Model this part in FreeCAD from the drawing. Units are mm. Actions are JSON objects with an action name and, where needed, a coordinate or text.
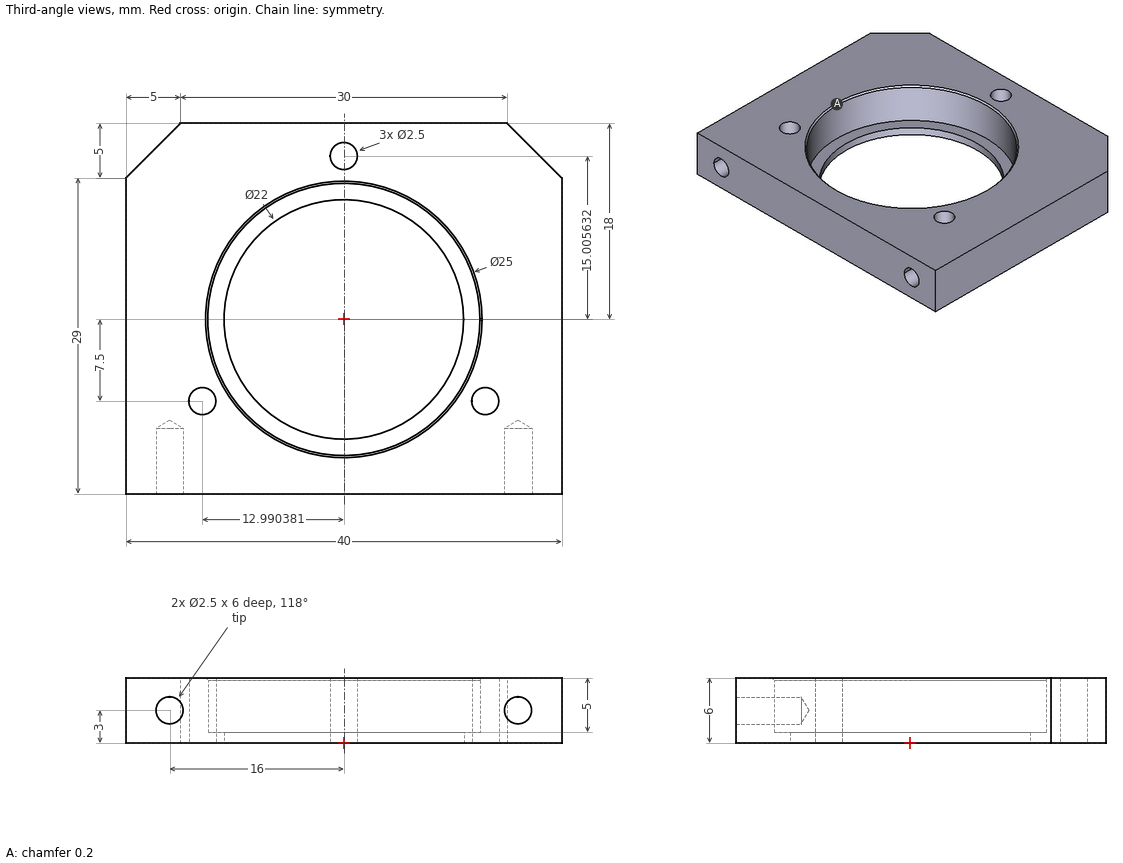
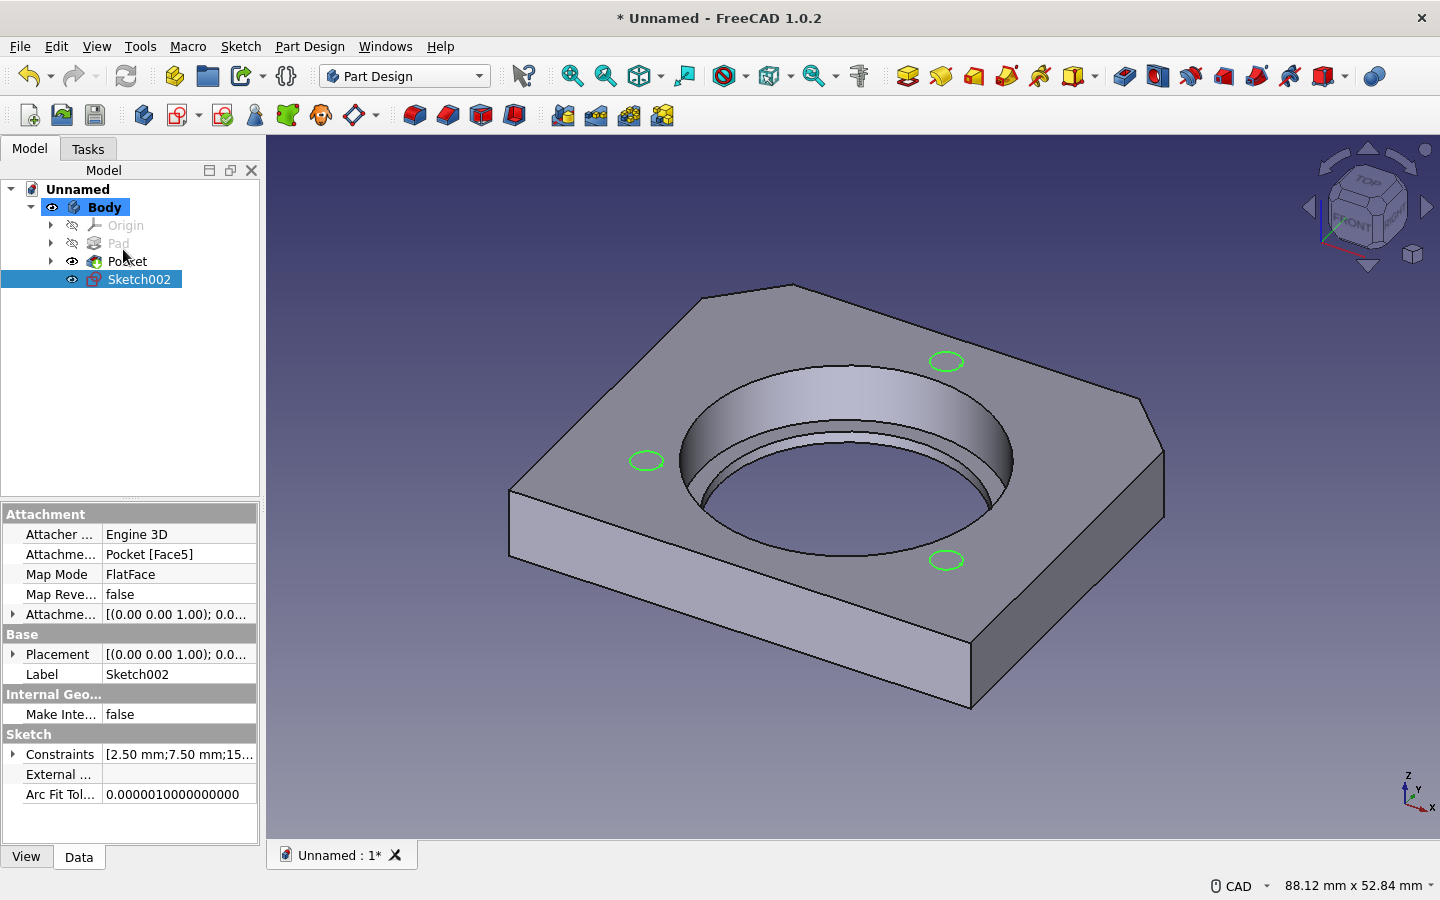
{"action": "left_click", "coordinate": [1125, 76]}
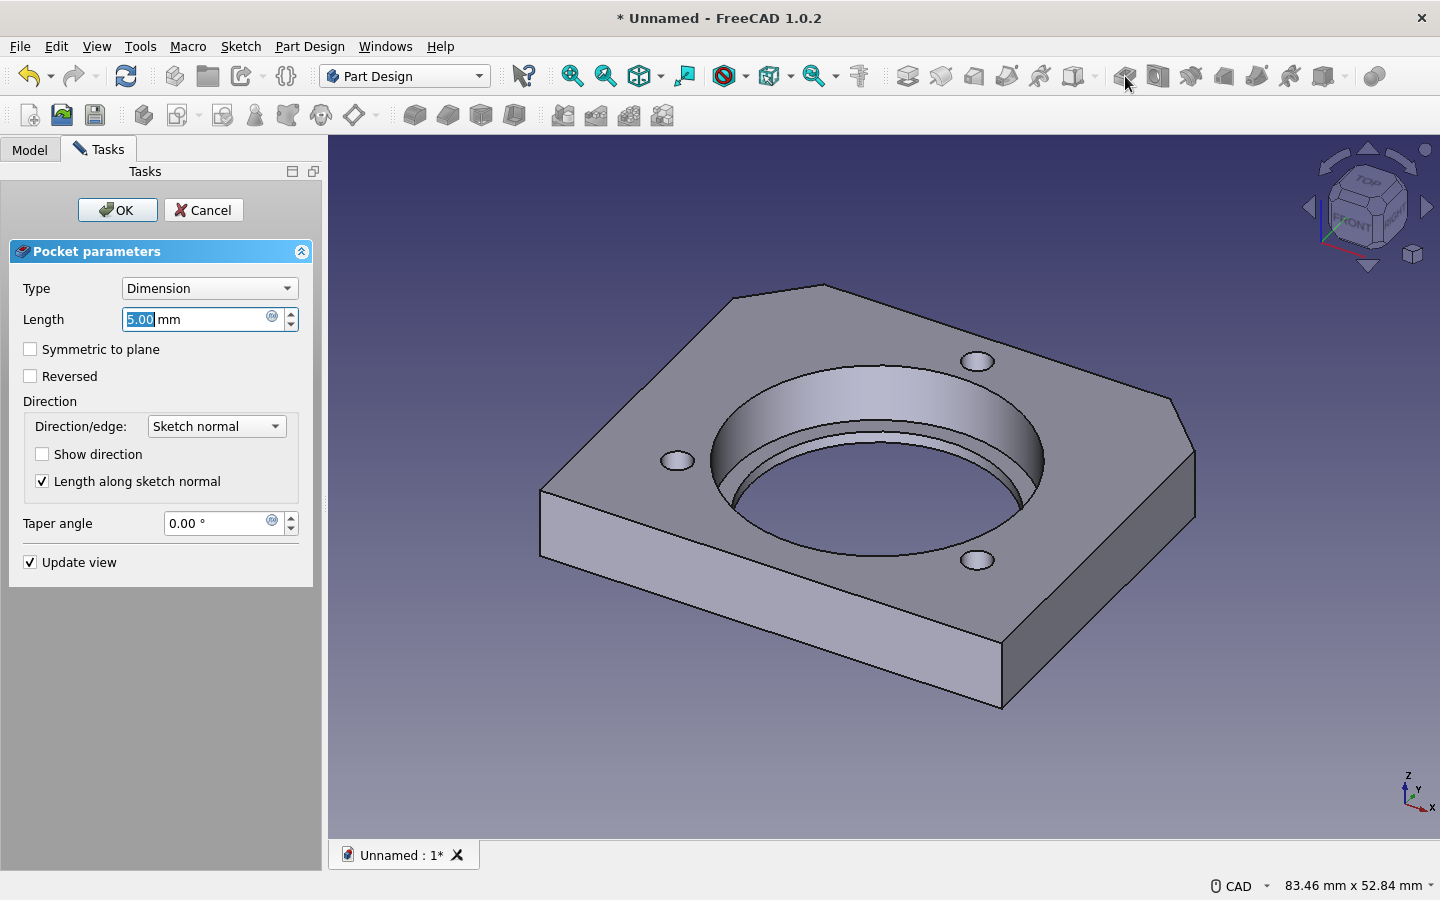
{"action": "left_click", "coordinate": [210, 288]}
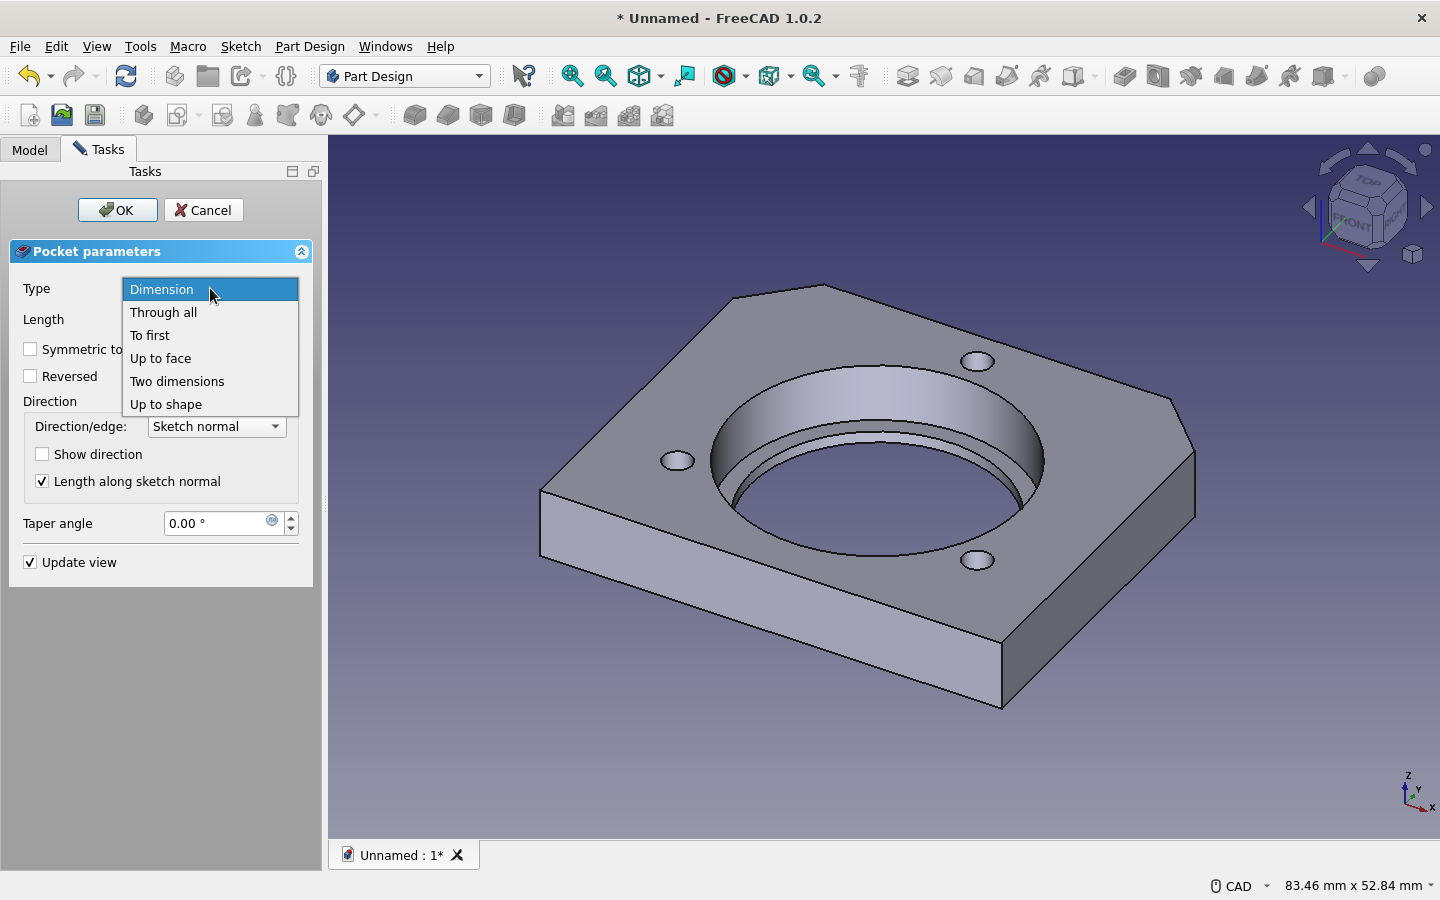
{"action": "left_click", "coordinate": [208, 312]}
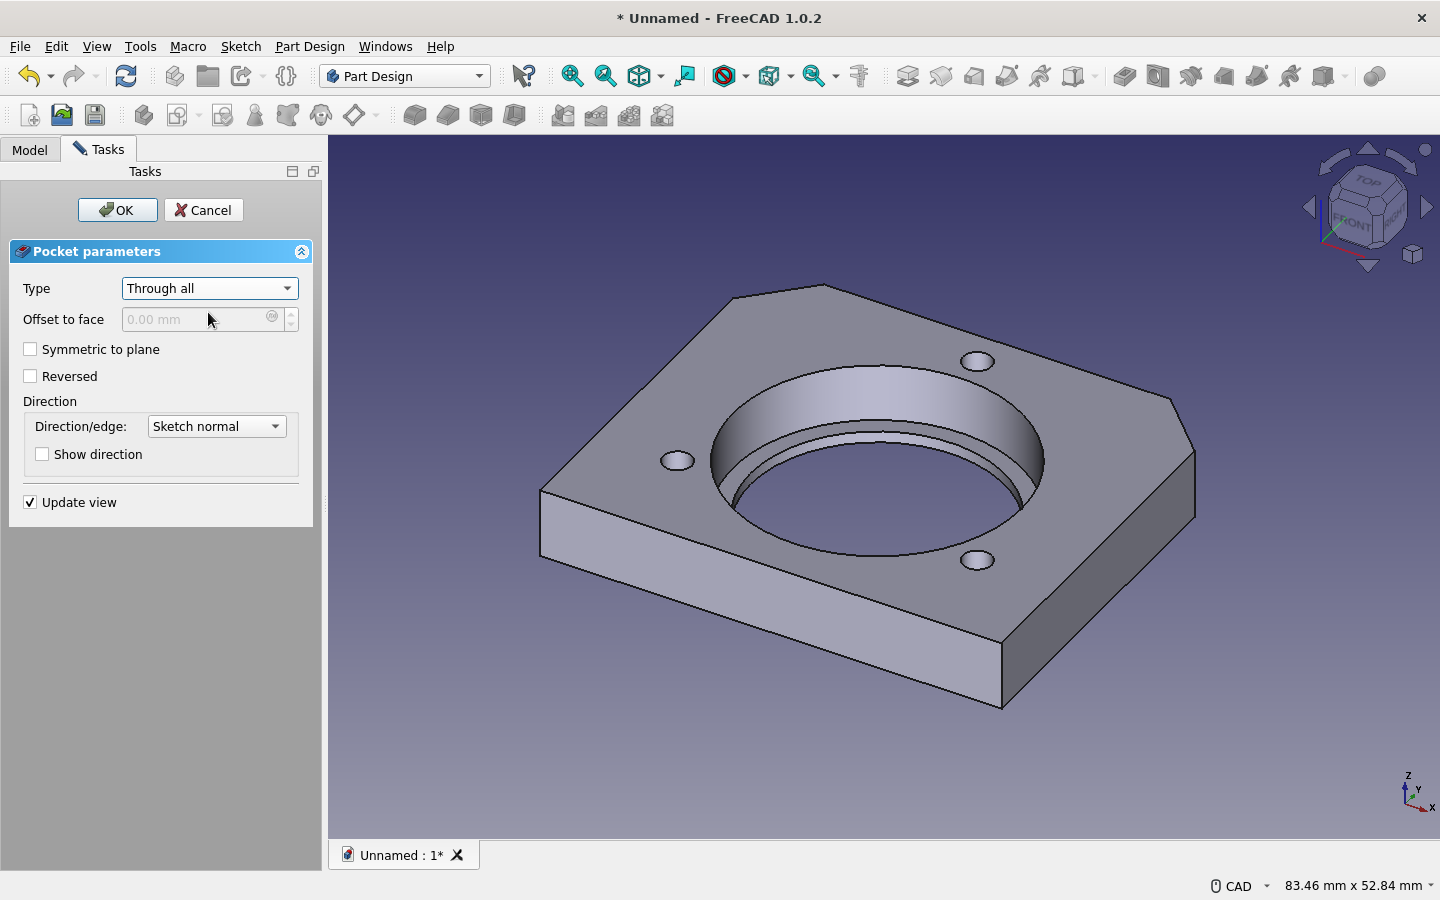
{"action": "left_click", "coordinate": [118, 210]}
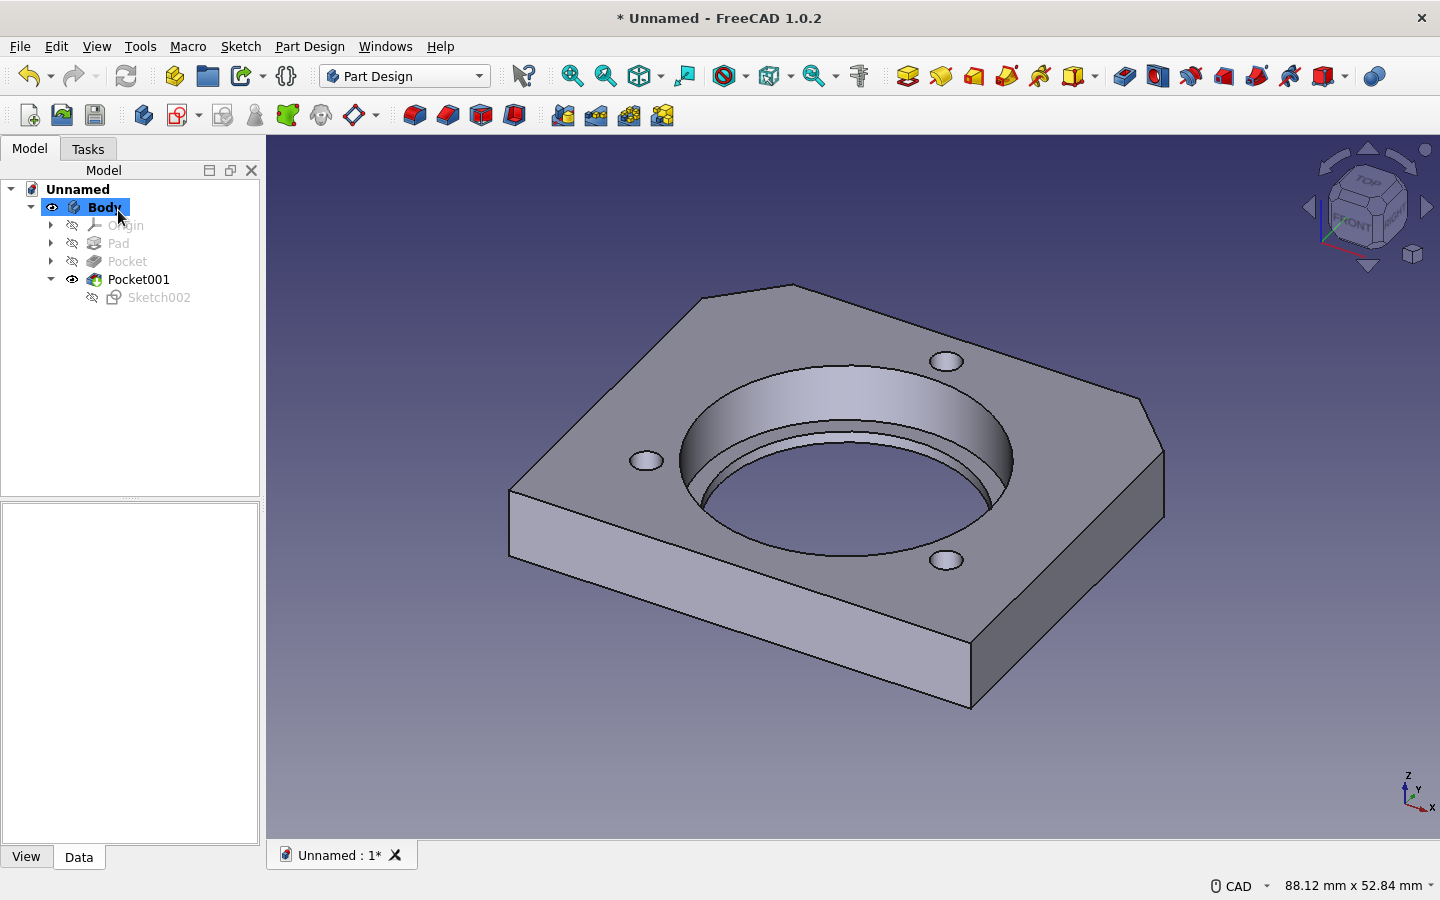
{"action": "left_click", "coordinate": [872, 642]}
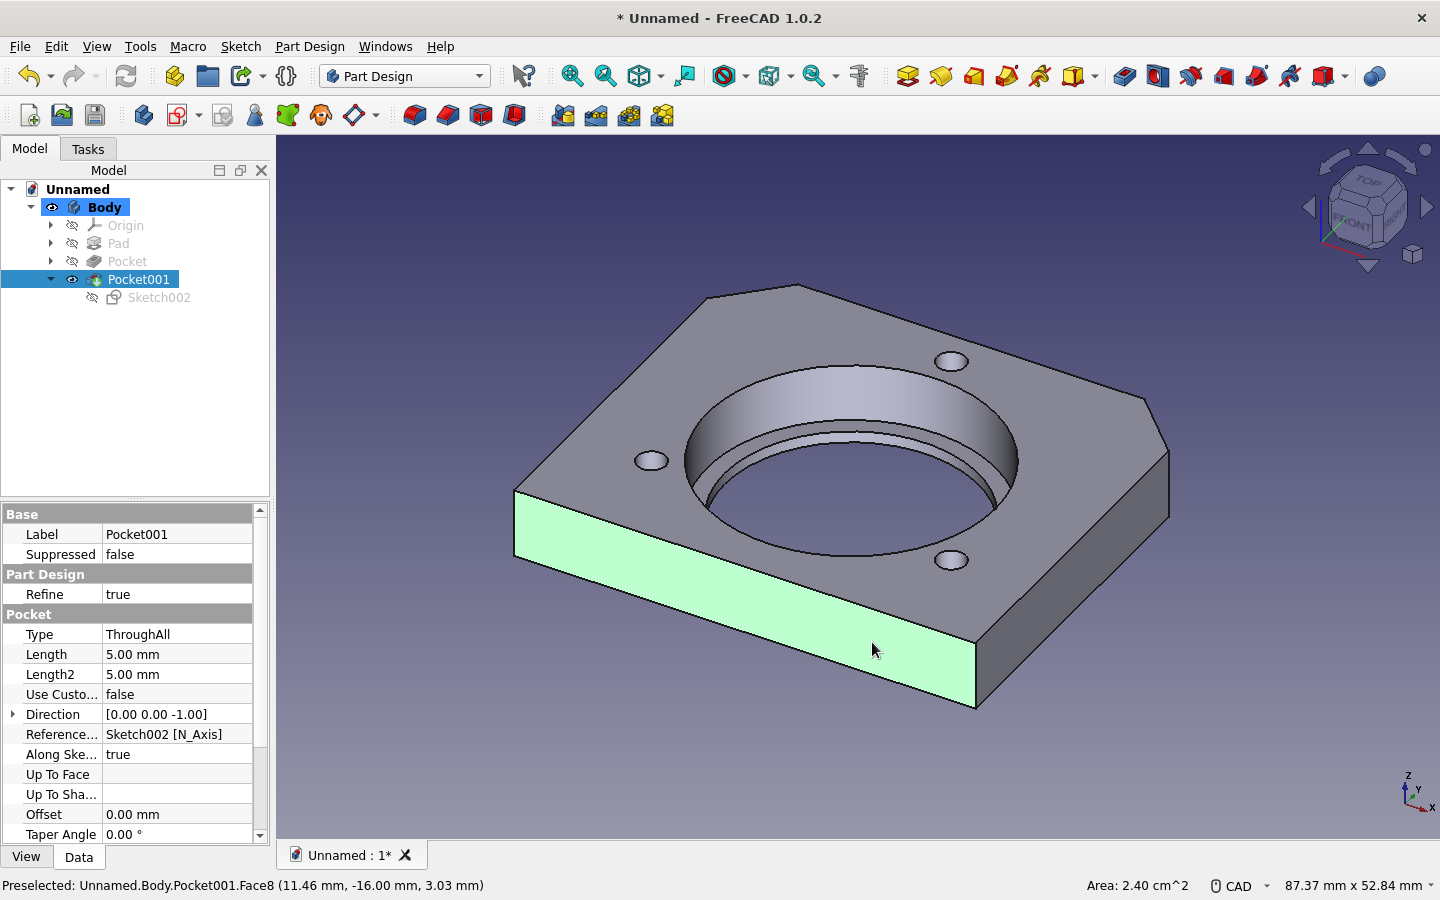
{"action": "left_click", "coordinate": [176, 116]}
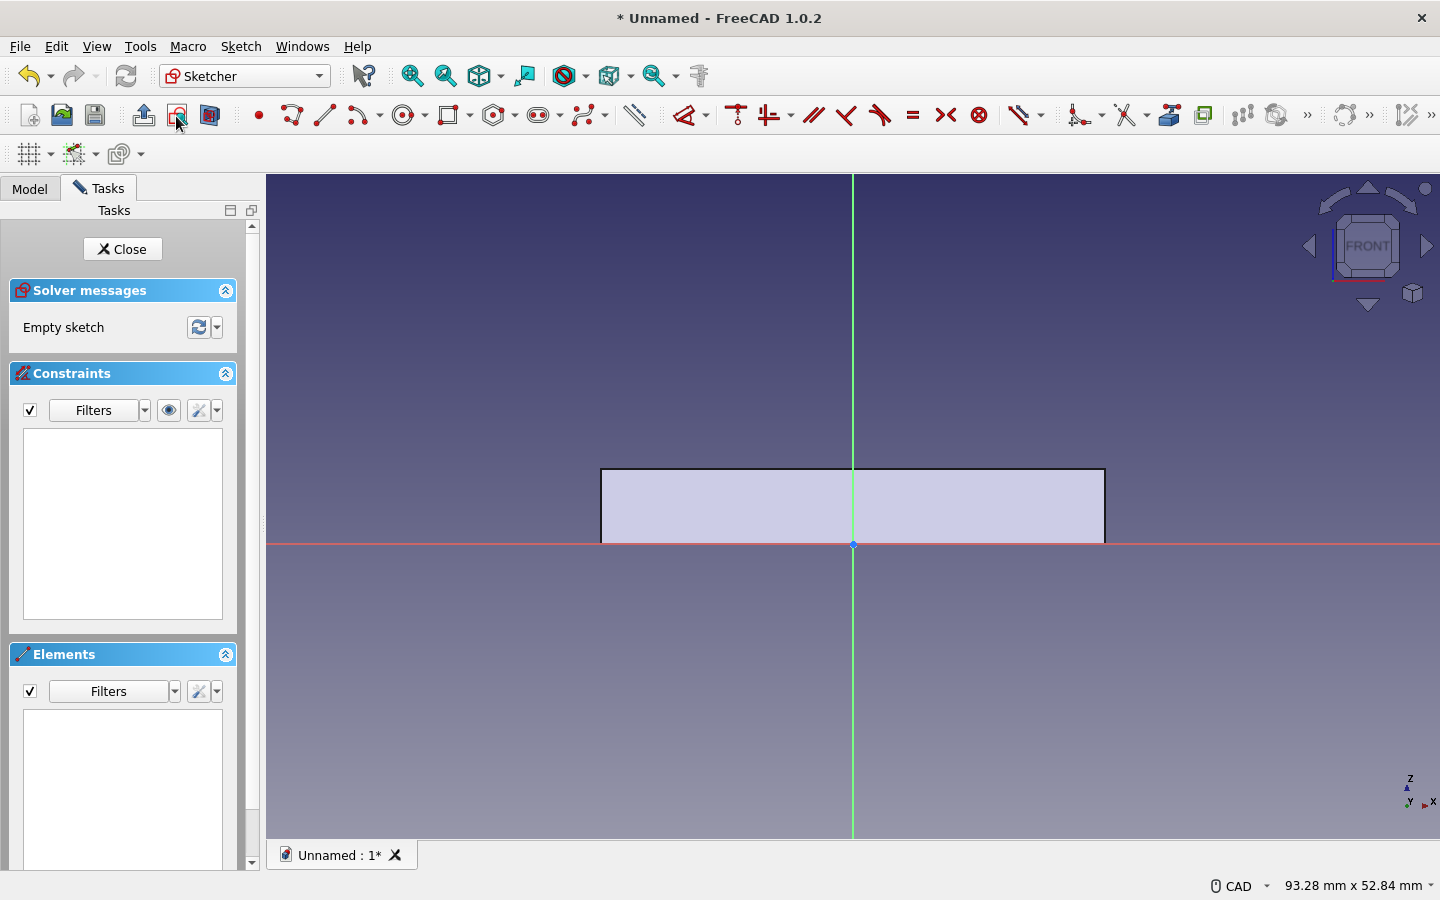
{"action": "scroll", "coordinate": [992, 540], "scroll_direction": "up", "scroll_amount": 2}